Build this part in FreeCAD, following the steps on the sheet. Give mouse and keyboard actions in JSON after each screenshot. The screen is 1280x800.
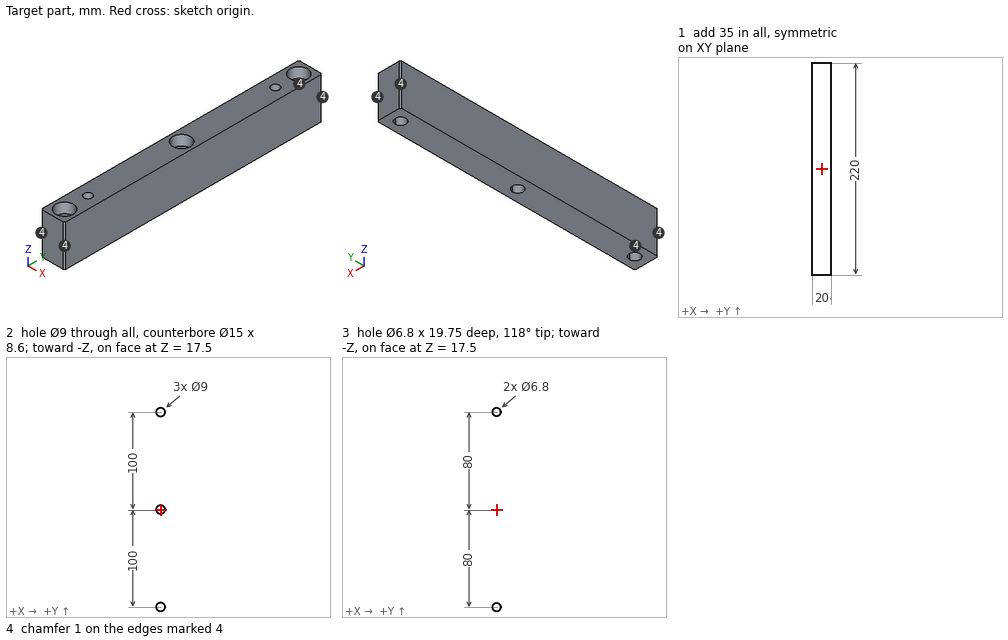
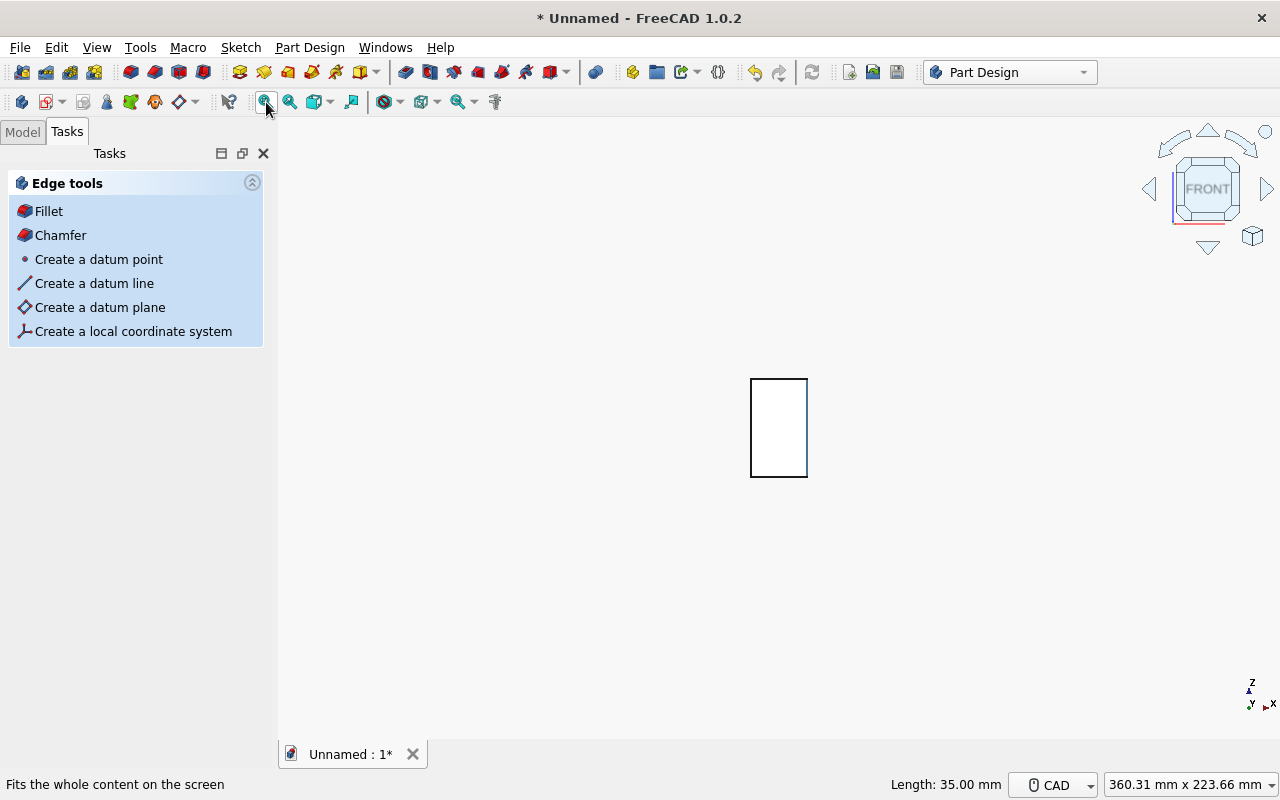
{"action": "left_click", "coordinate": [751, 427], "text": "ctrl"}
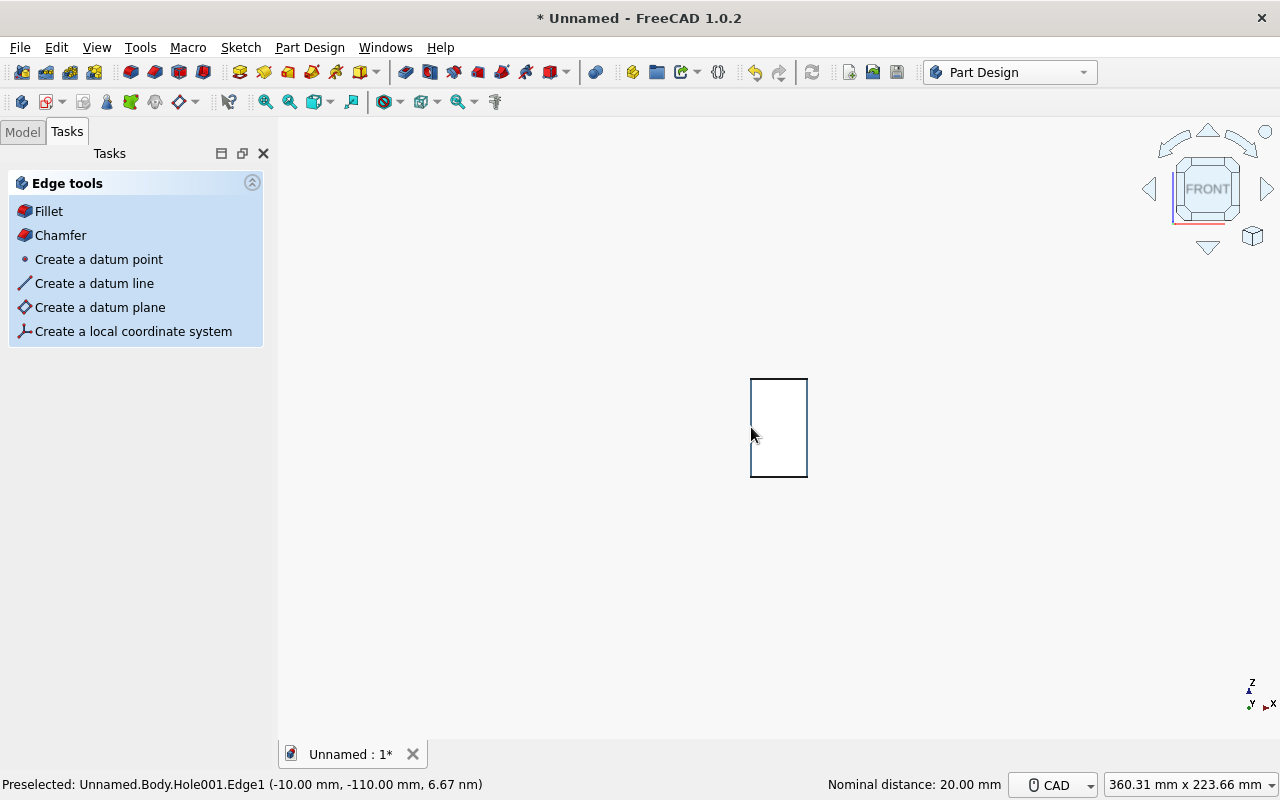
{"action": "key", "text": "3"}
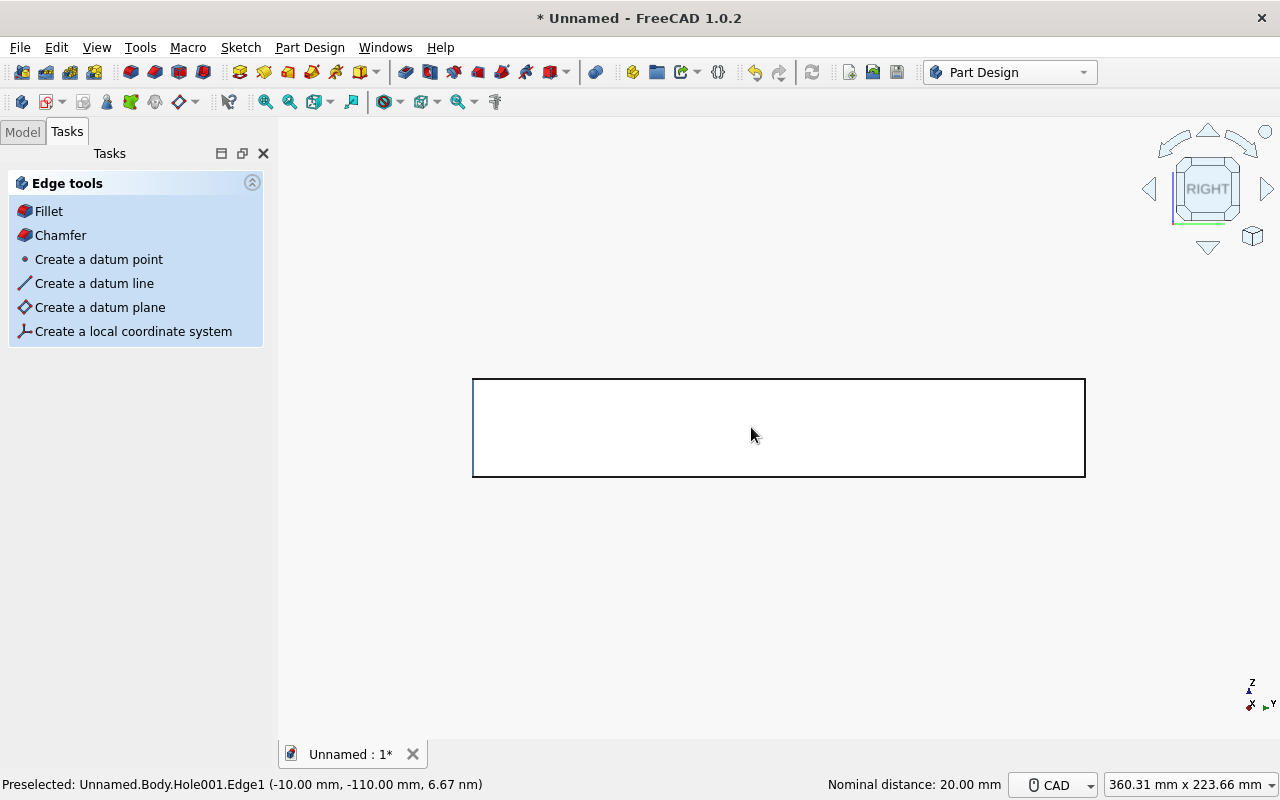
{"action": "left_click", "coordinate": [1085, 427], "text": "ctrl"}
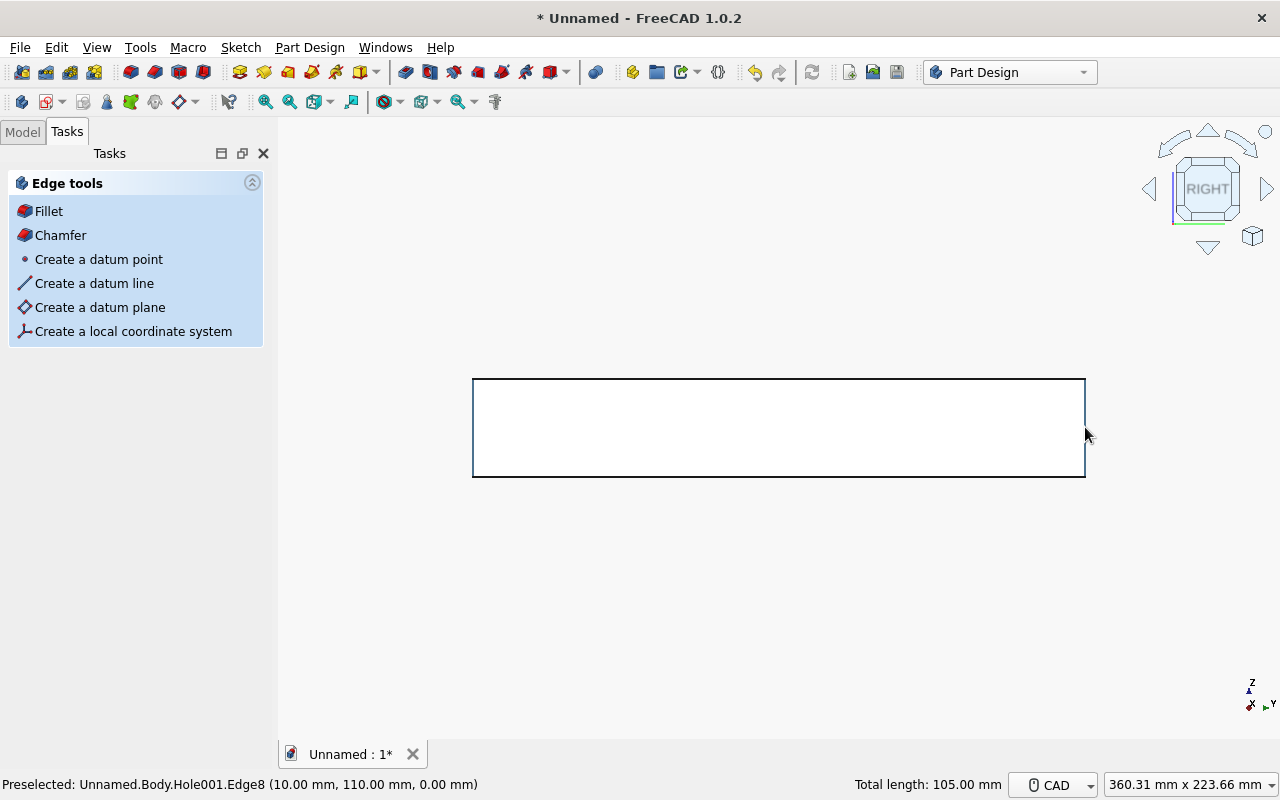
{"action": "key", "text": "5"}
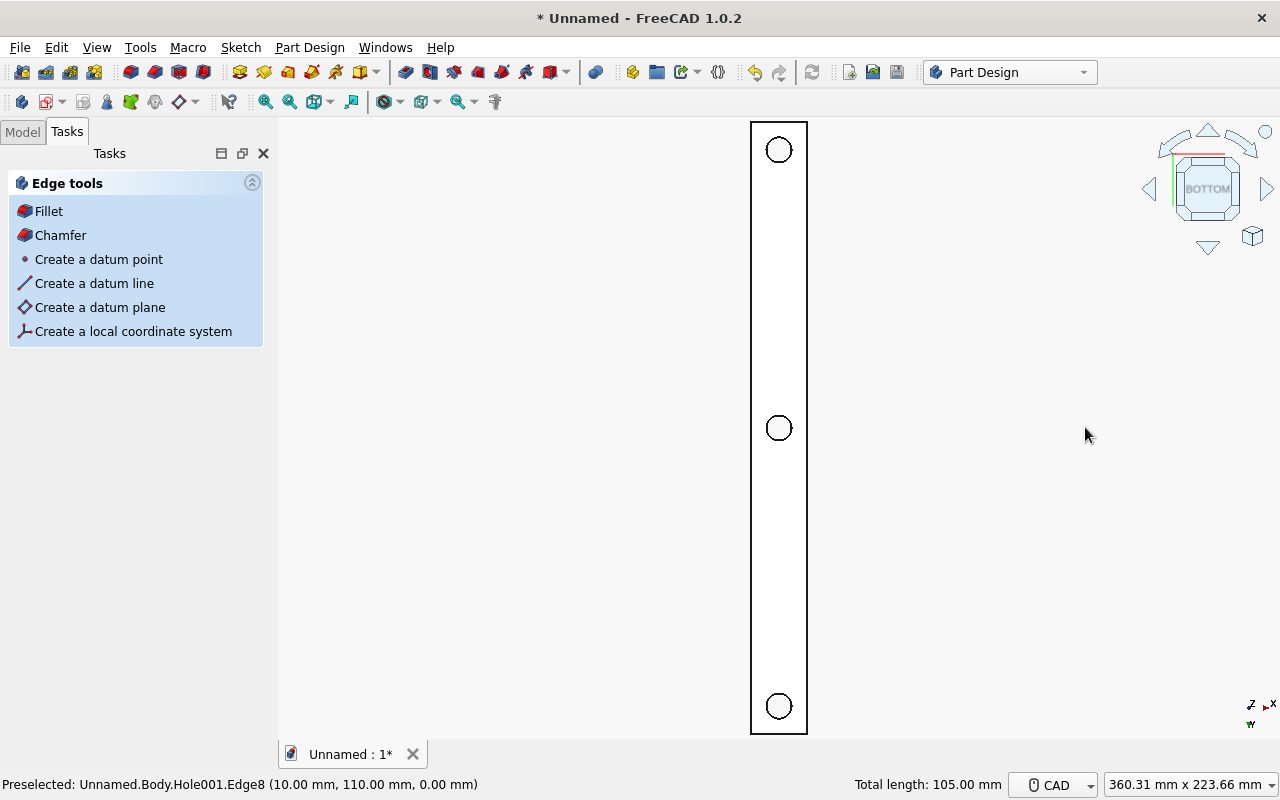
{"action": "key", "text": "4"}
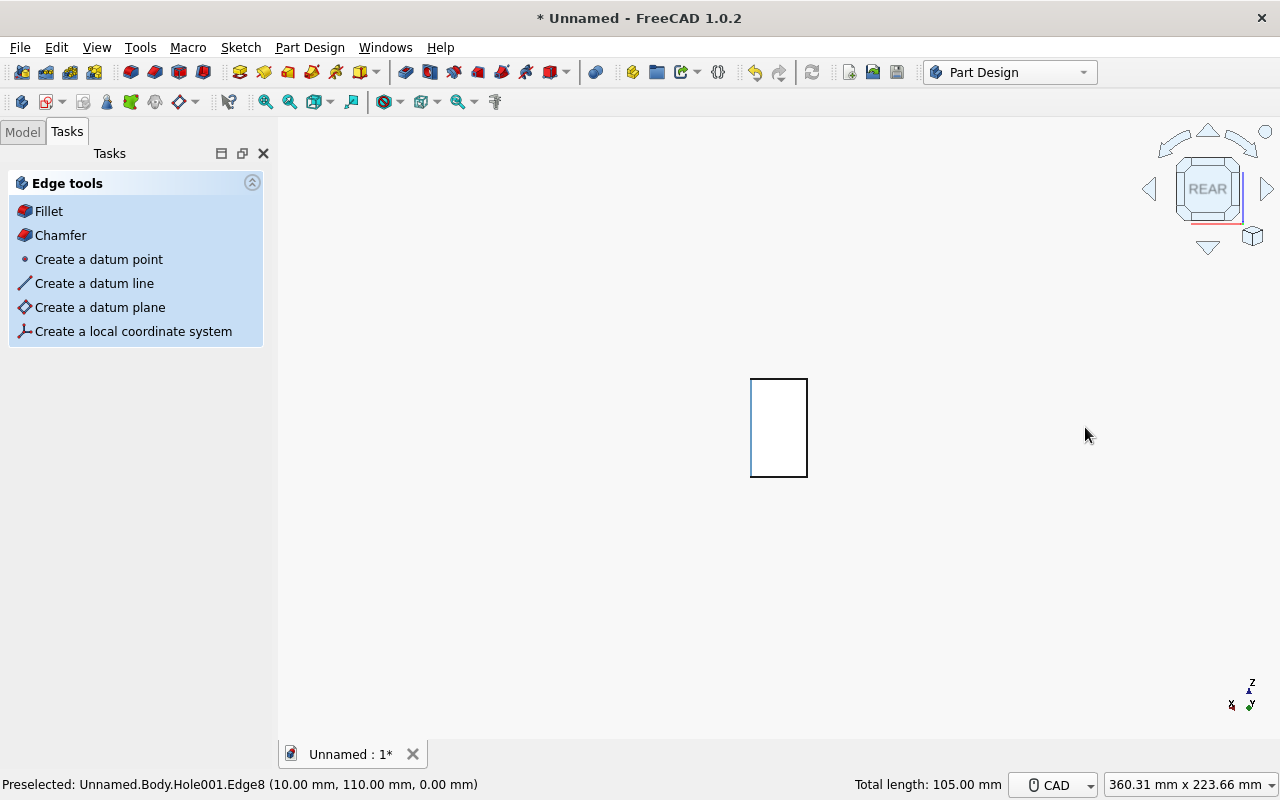
{"action": "key", "text": "v f"}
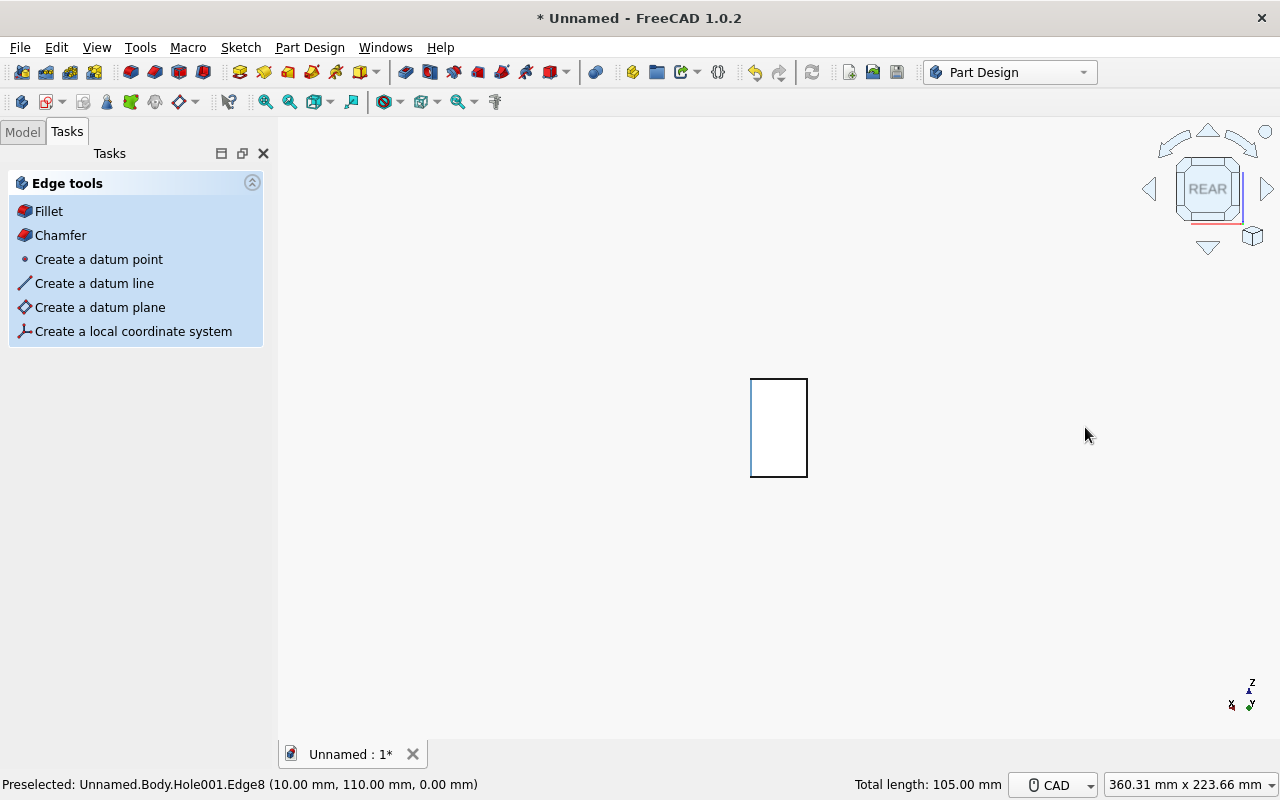
{"action": "left_click", "coordinate": [807, 427], "text": "ctrl"}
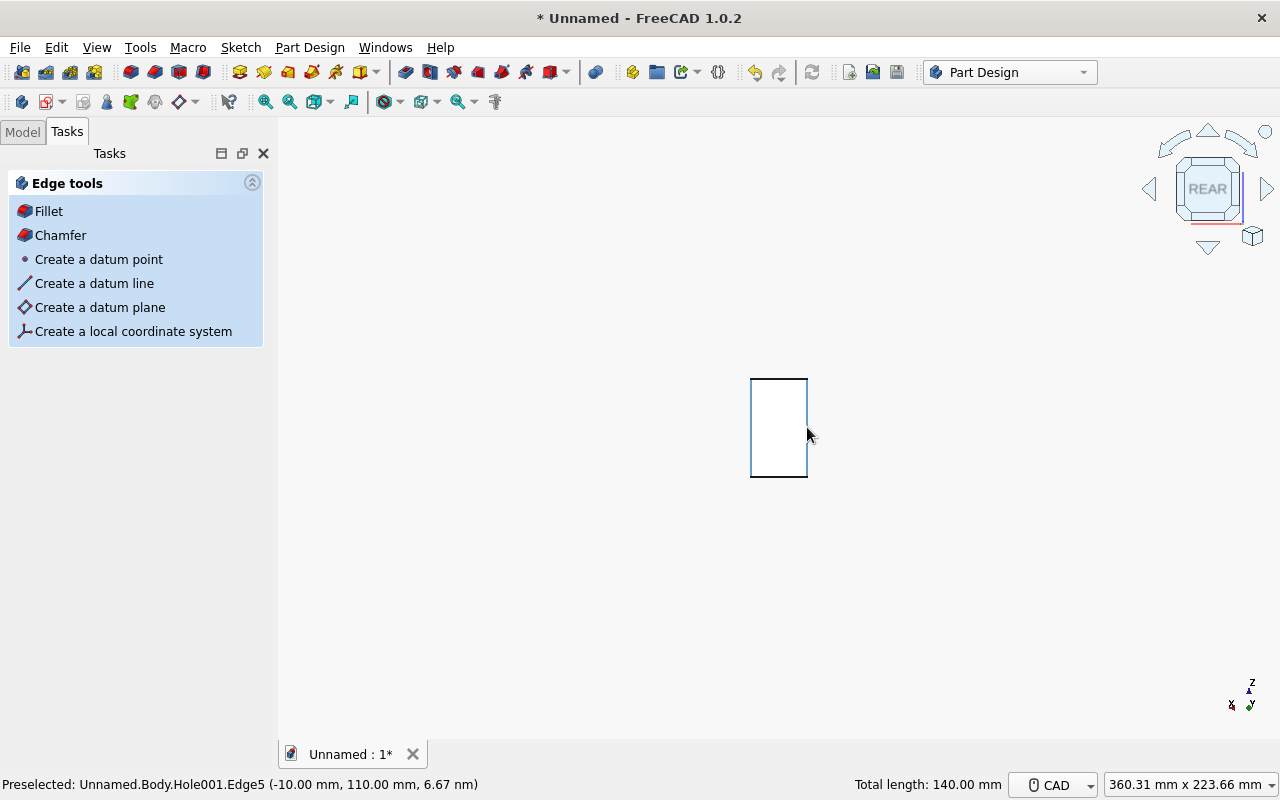
{"action": "left_click", "coordinate": [156, 72]}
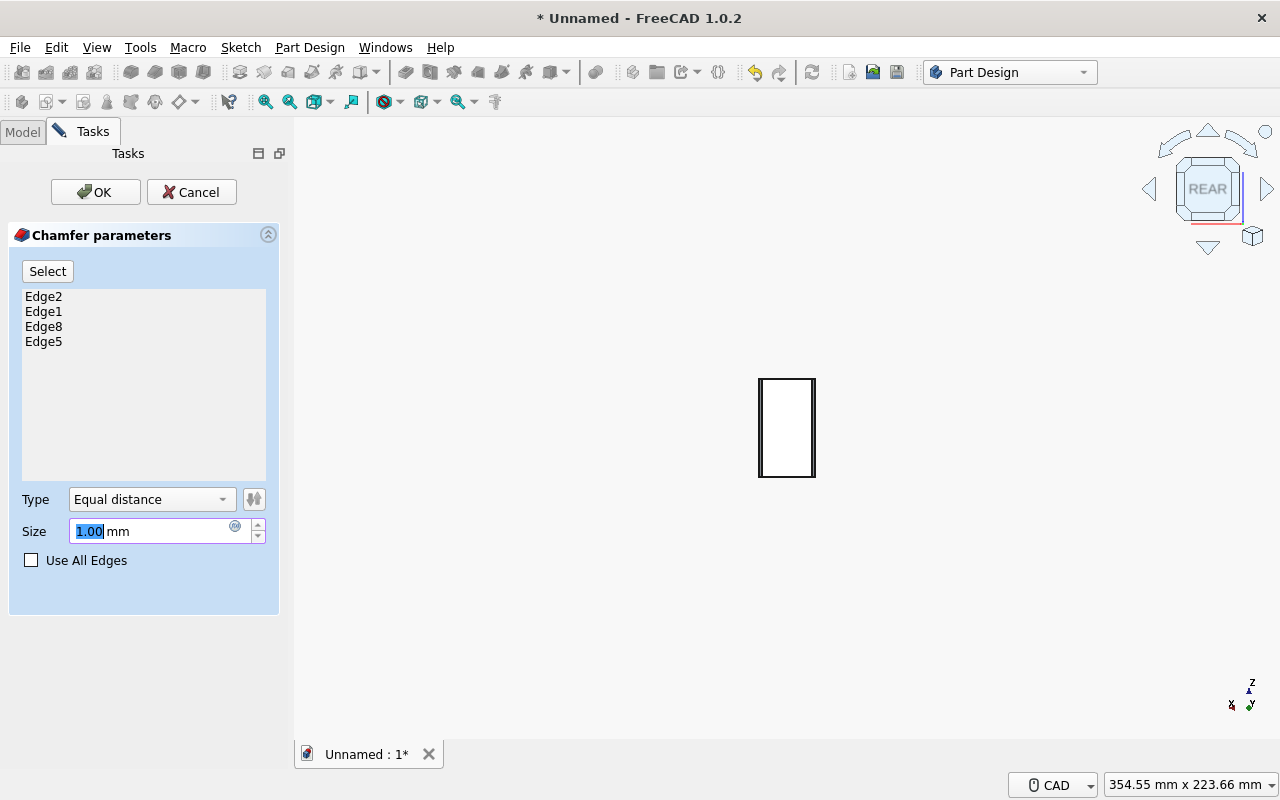
{"action": "type", "text": "1"}
{"action": "key", "text": "Tab"}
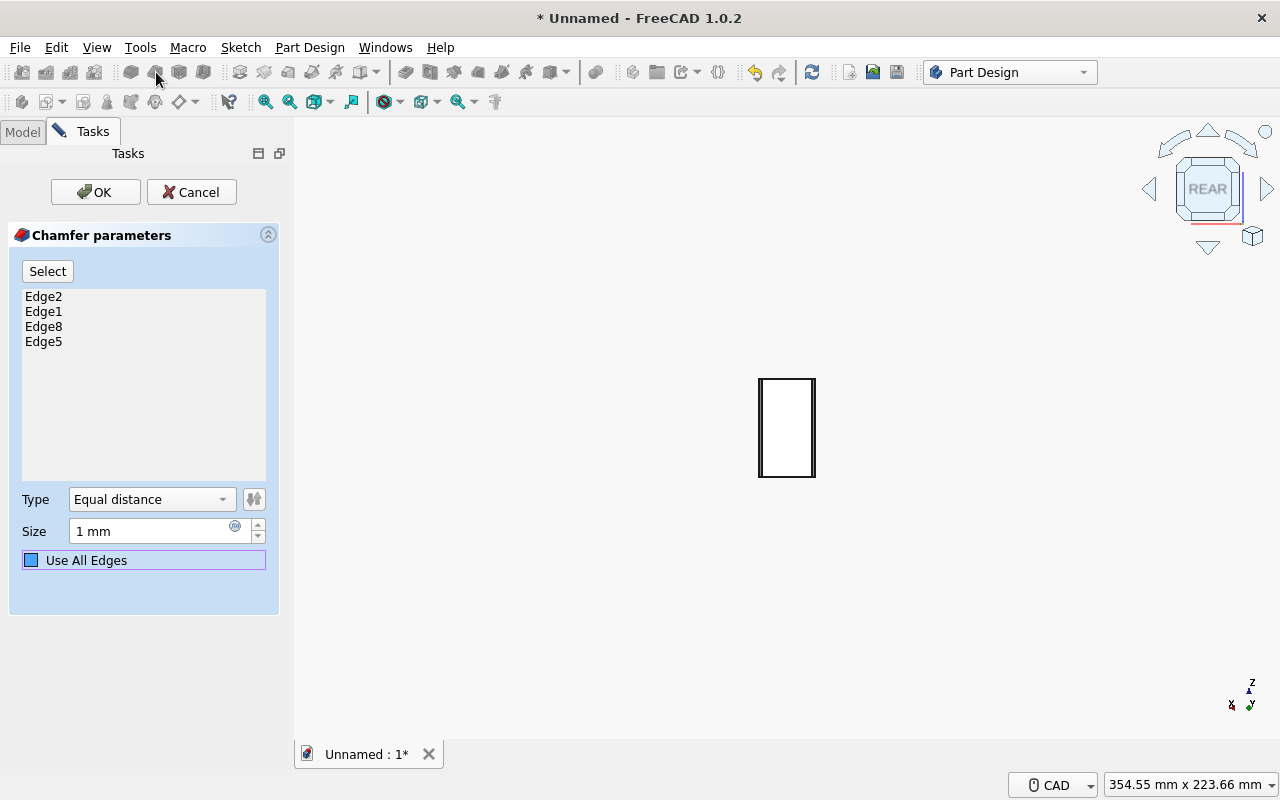
{"action": "left_click", "coordinate": [96, 192]}